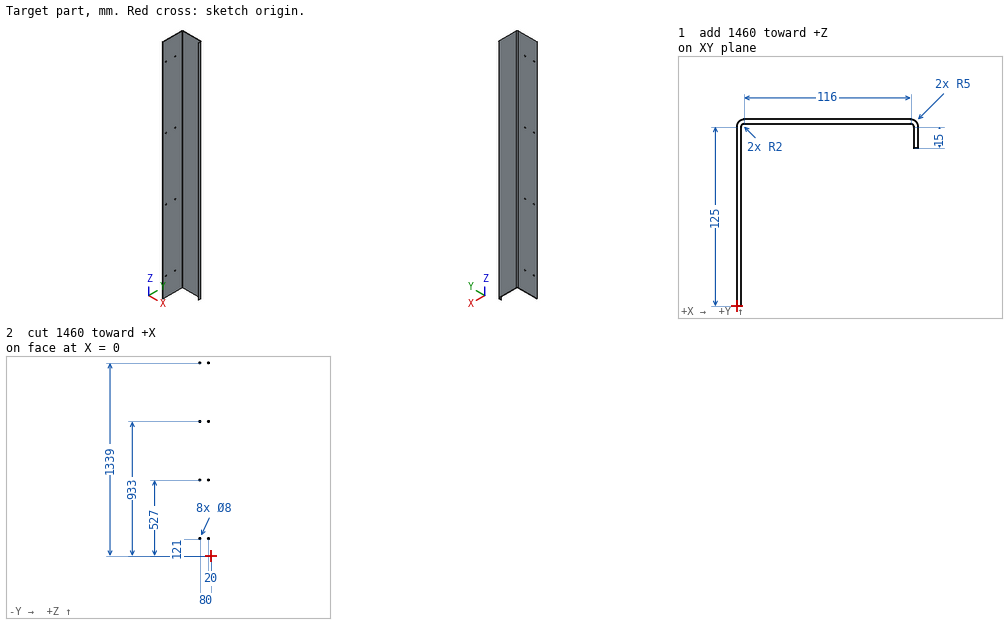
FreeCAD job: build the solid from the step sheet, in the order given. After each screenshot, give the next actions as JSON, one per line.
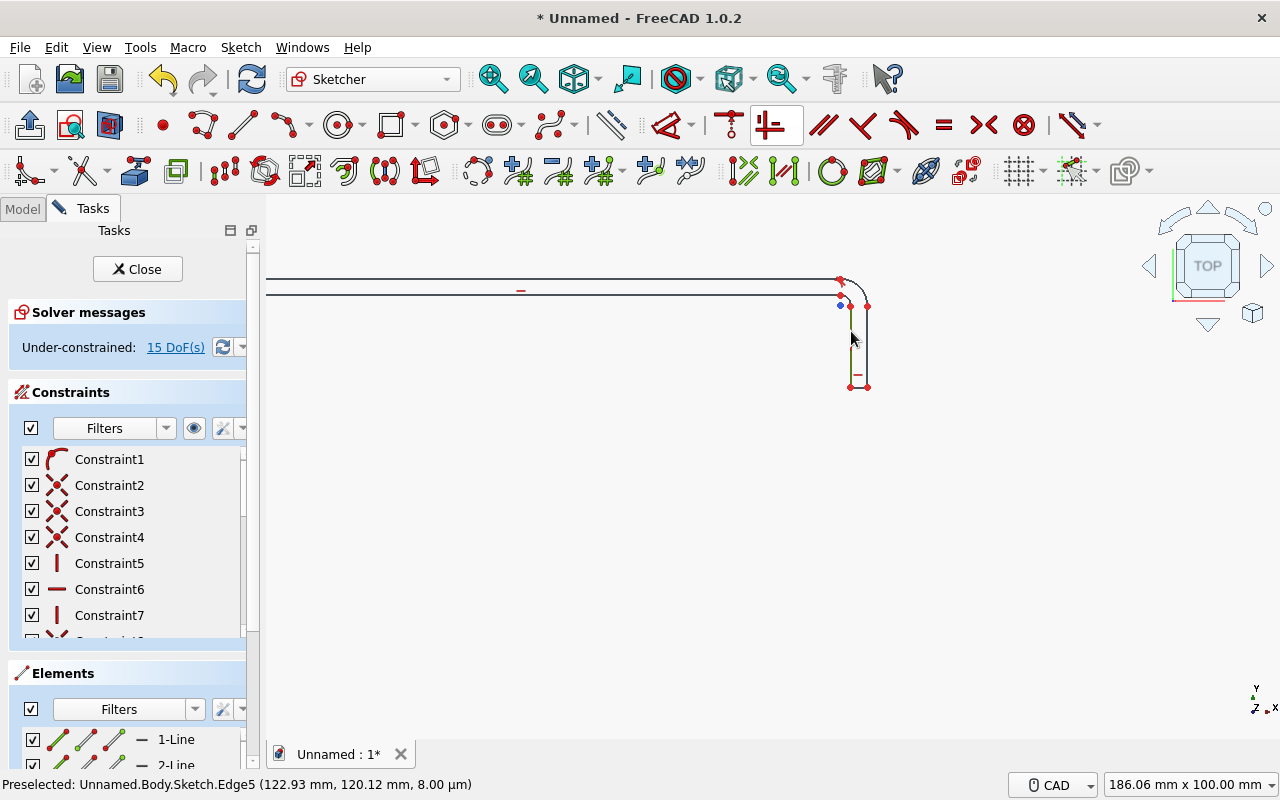
{"action": "scroll", "coordinate": [848, 298], "scroll_direction": "up", "scroll_amount": 3}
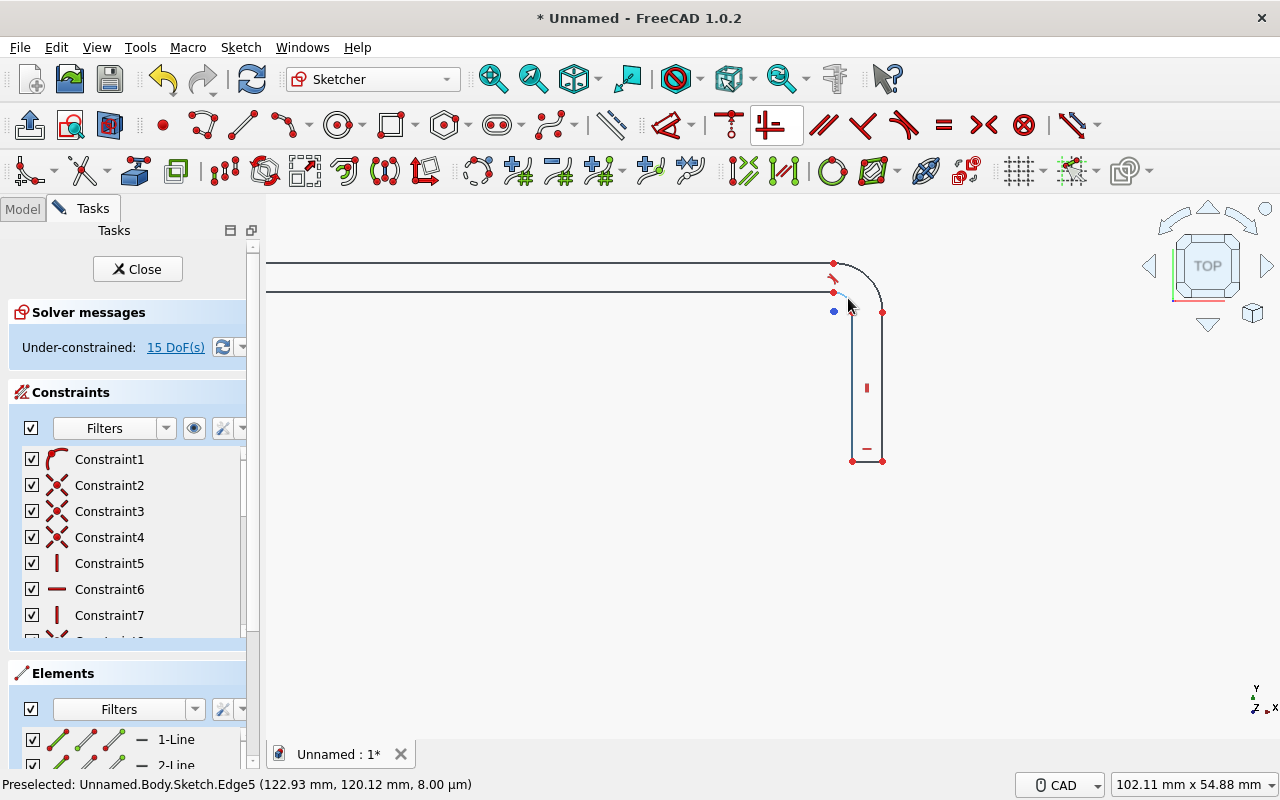
{"action": "left_click", "coordinate": [847, 298]}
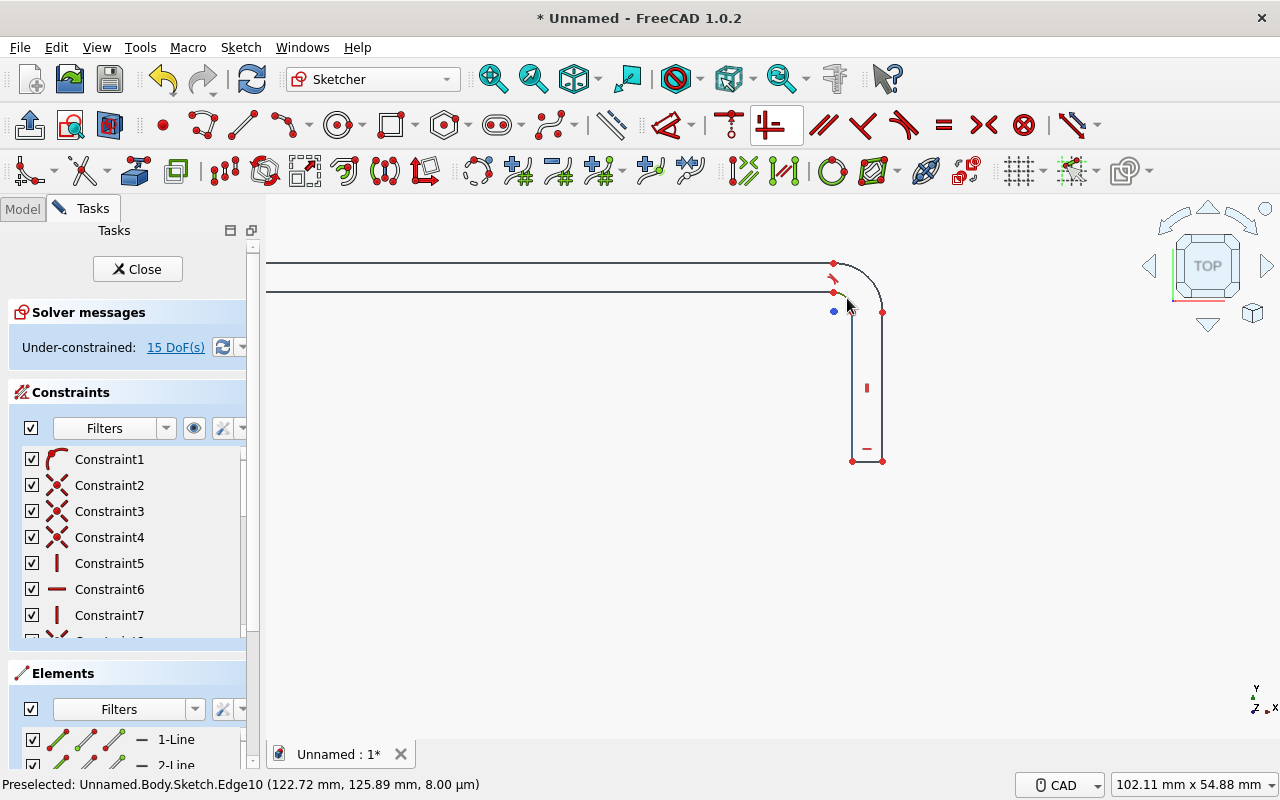
{"action": "left_click", "coordinate": [904, 126]}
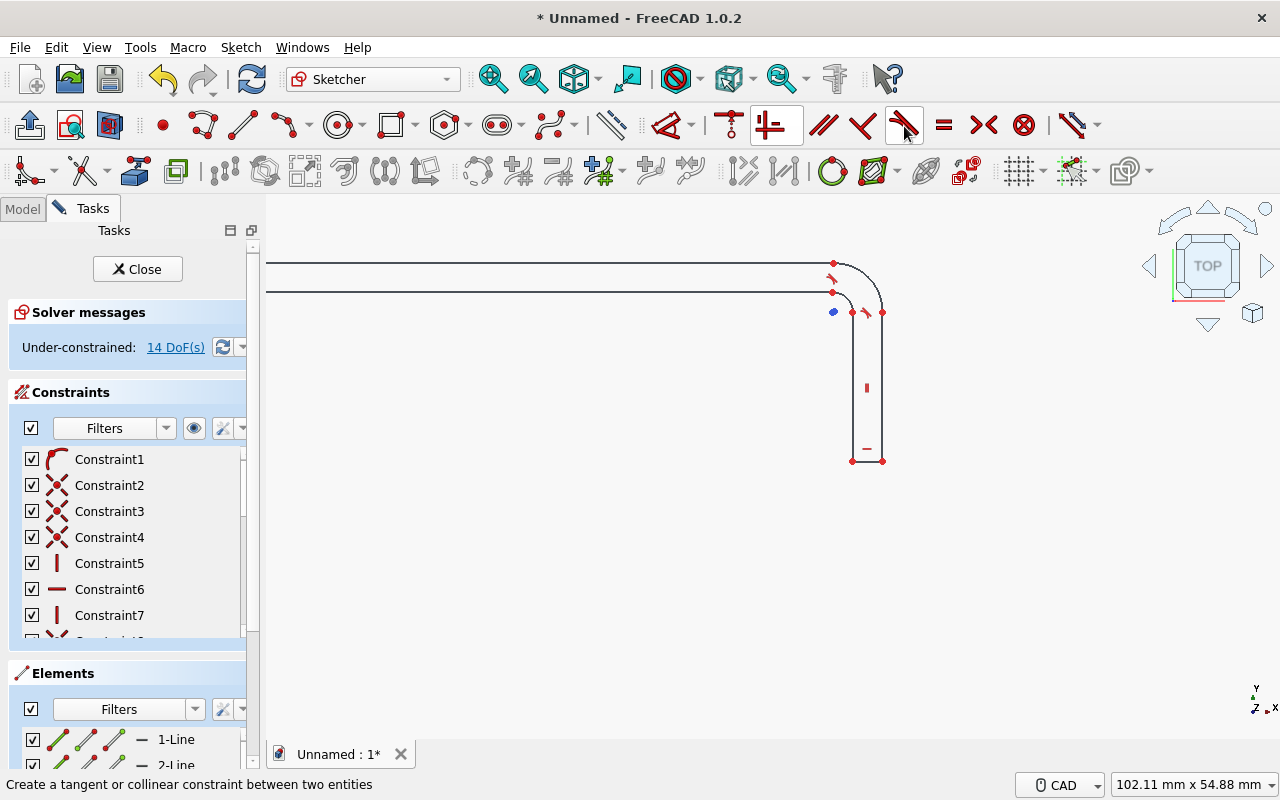
{"action": "left_click", "coordinate": [882, 417]}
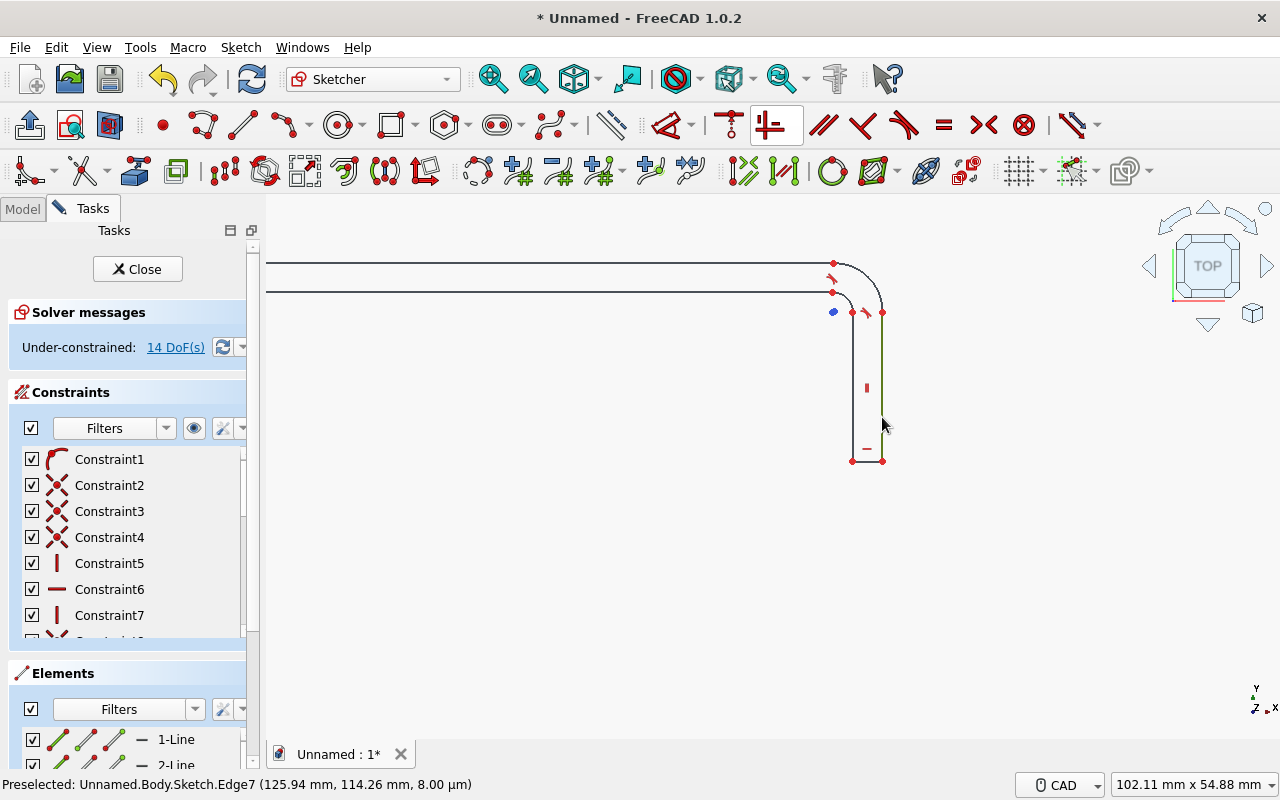
{"action": "left_click", "coordinate": [877, 290]}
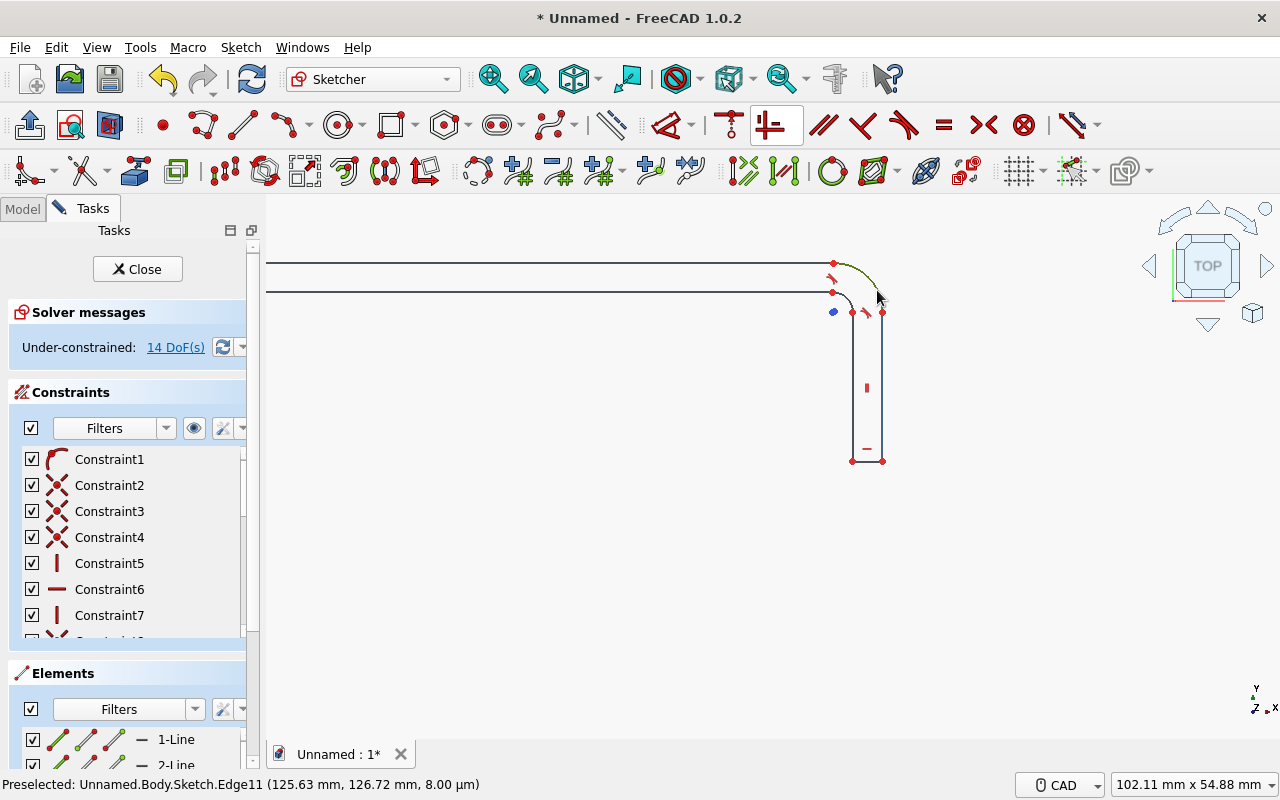
{"action": "left_click", "coordinate": [904, 126]}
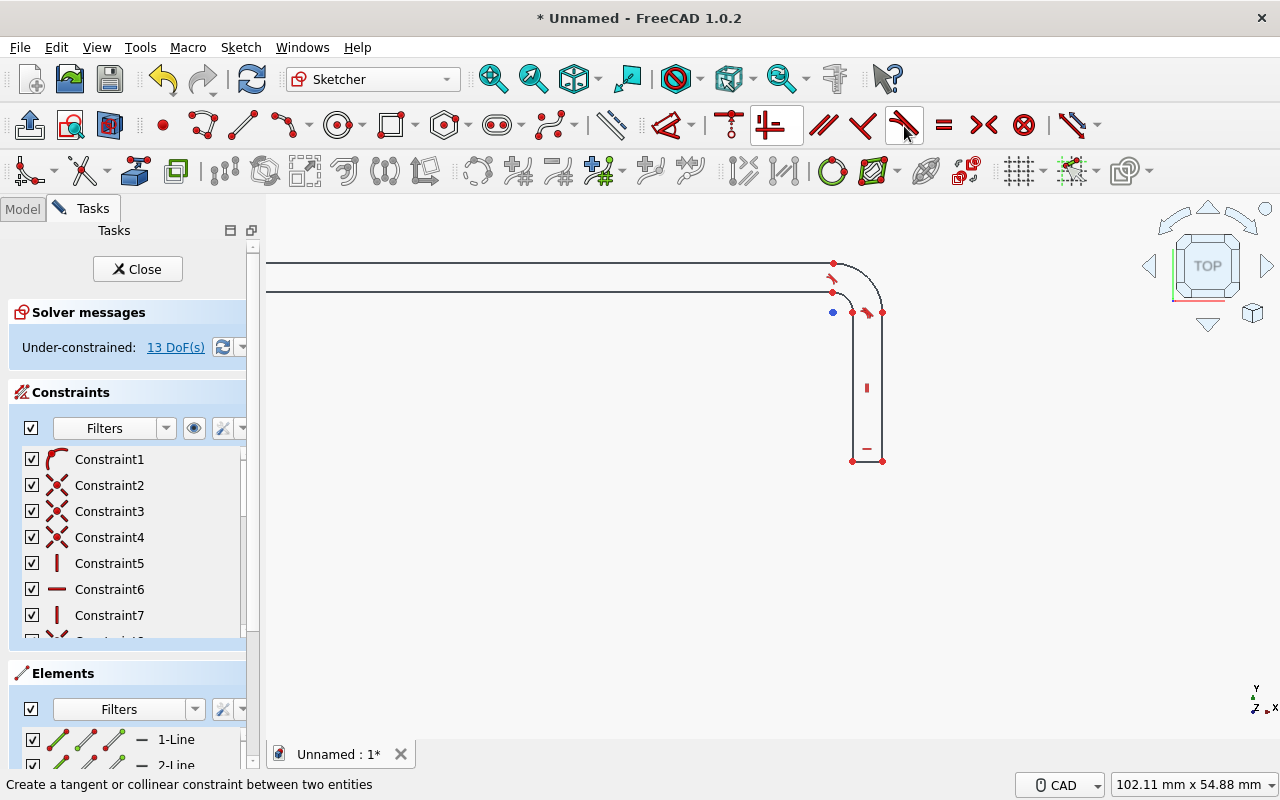
{"action": "left_click", "coordinate": [487, 263]}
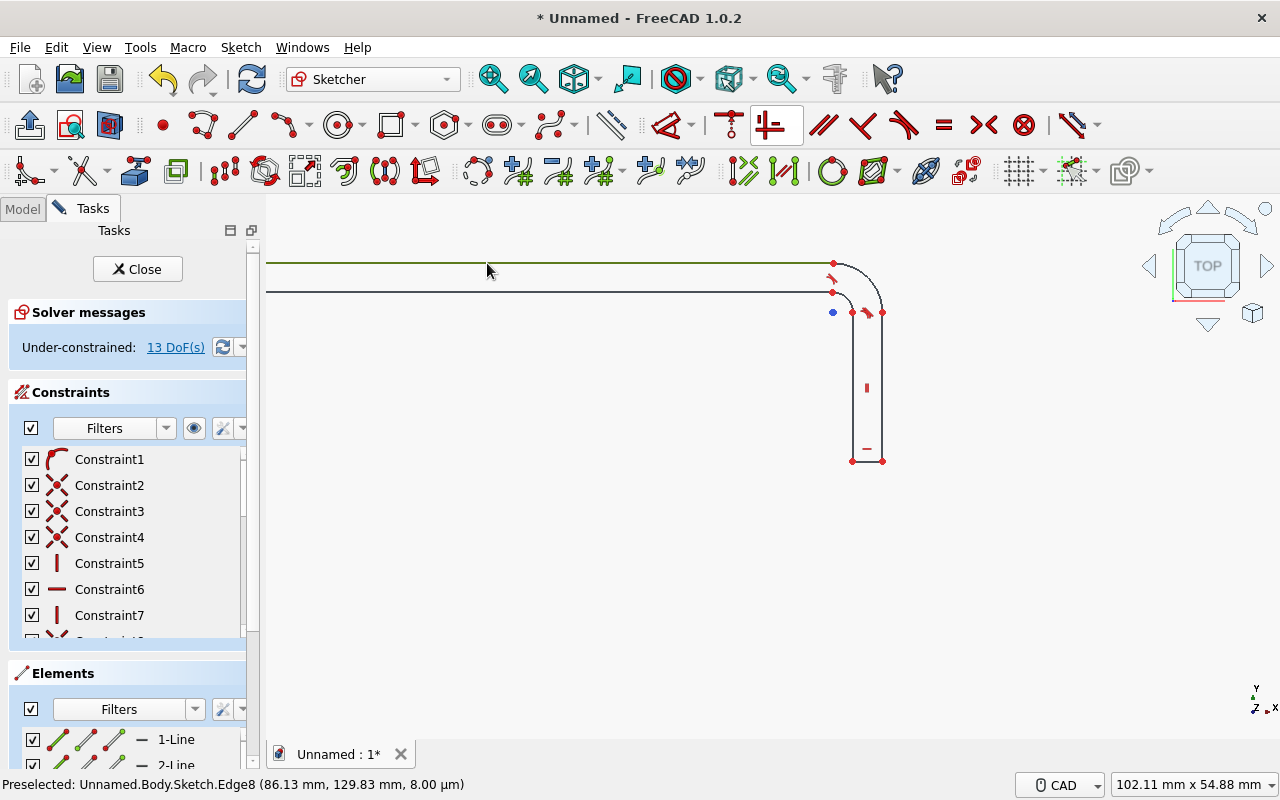
{"action": "left_click", "coordinate": [877, 290]}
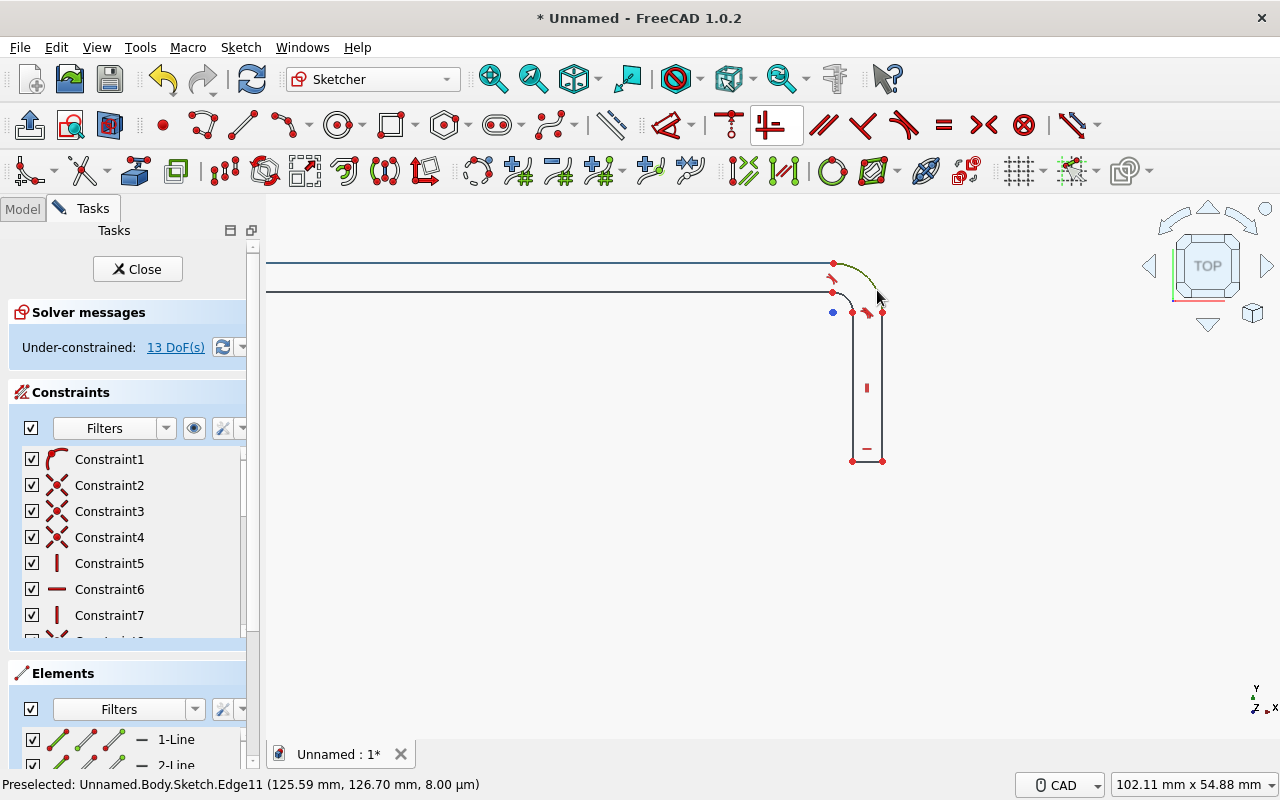
{"action": "left_click", "coordinate": [904, 126]}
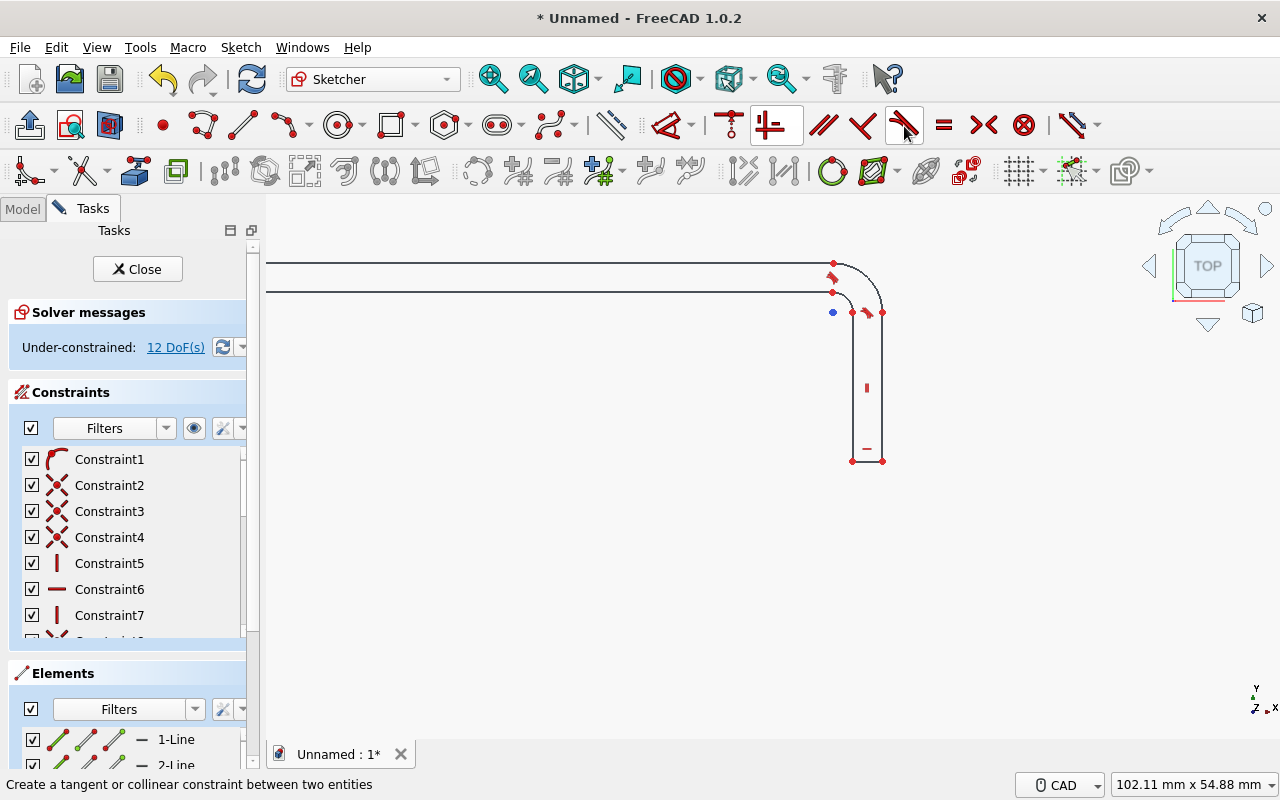
{"action": "left_click", "coordinate": [487, 263]}